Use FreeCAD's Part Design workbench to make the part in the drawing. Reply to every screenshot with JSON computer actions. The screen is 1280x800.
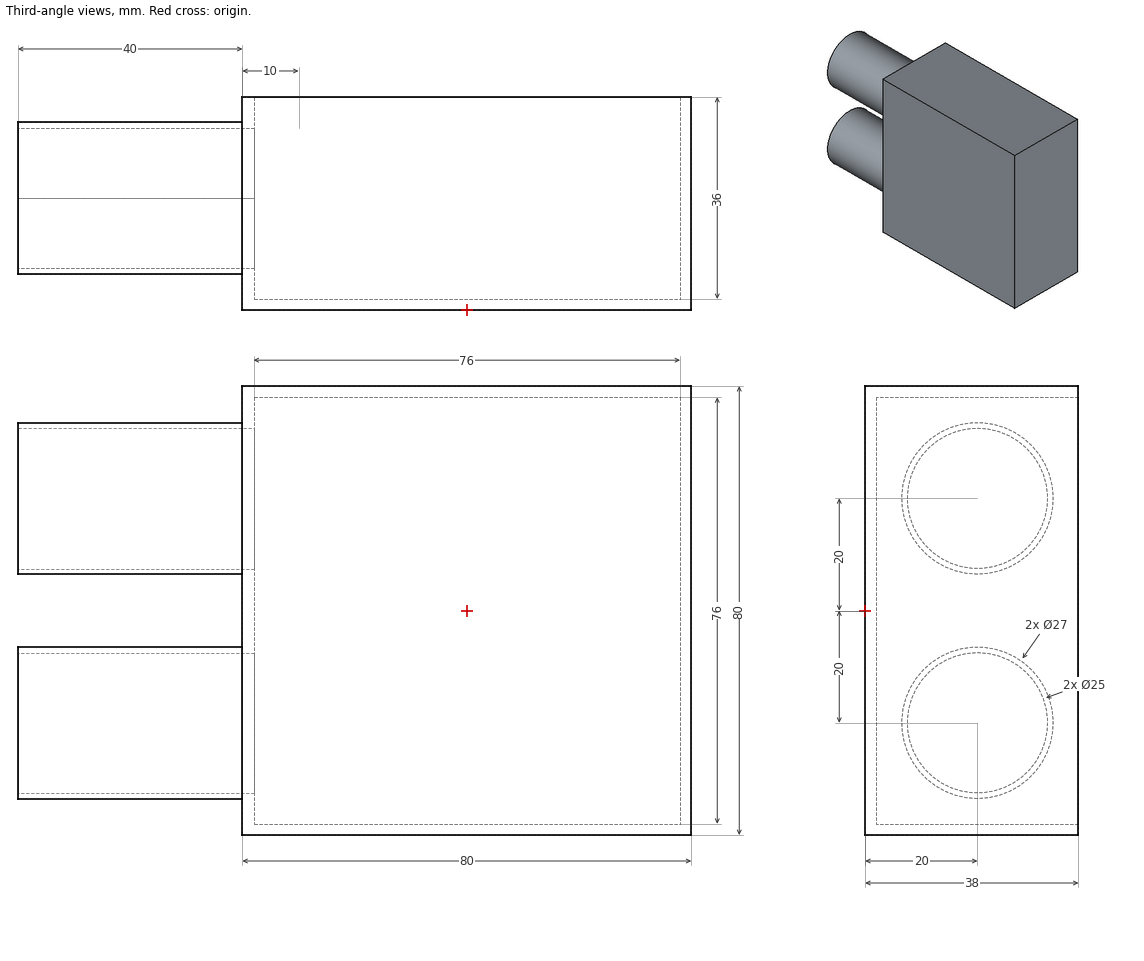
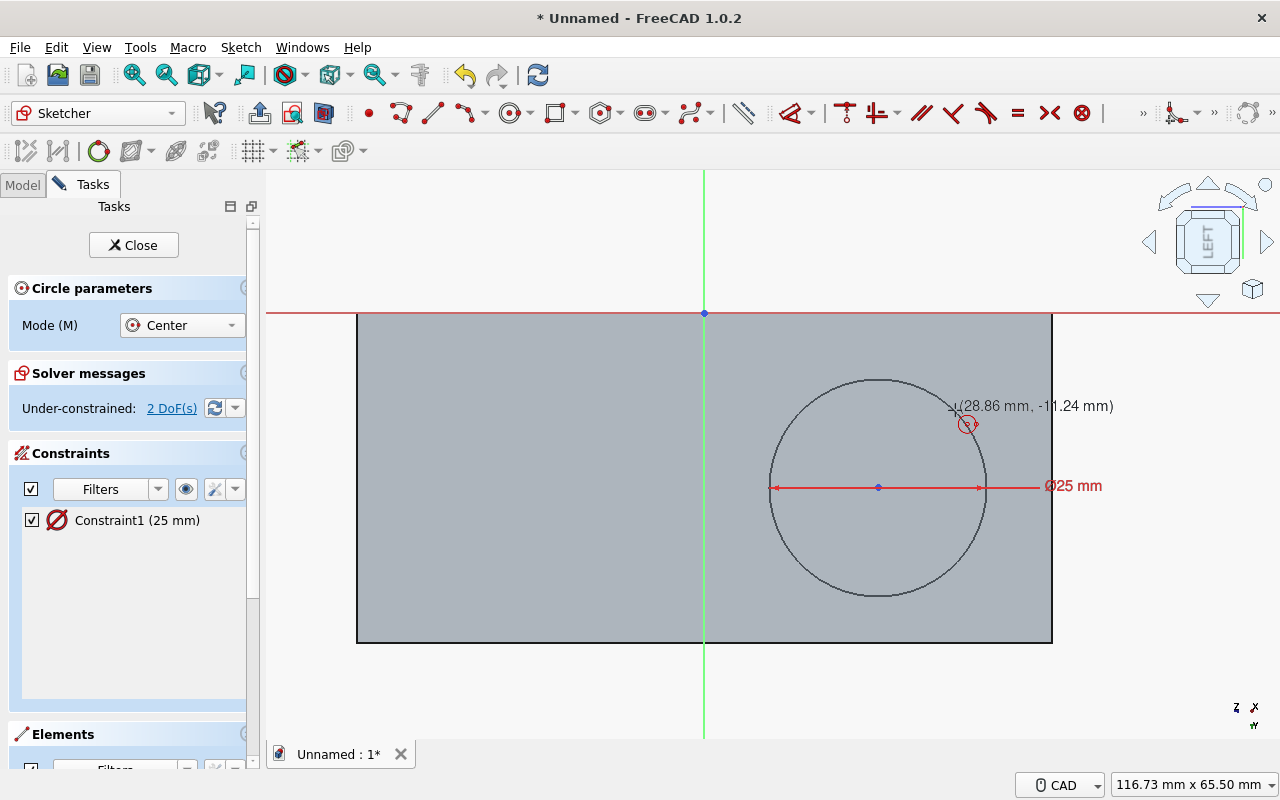
{"action": "left_click", "coordinate": [531, 487]}
{"action": "mouse_move", "coordinate": [607, 410]}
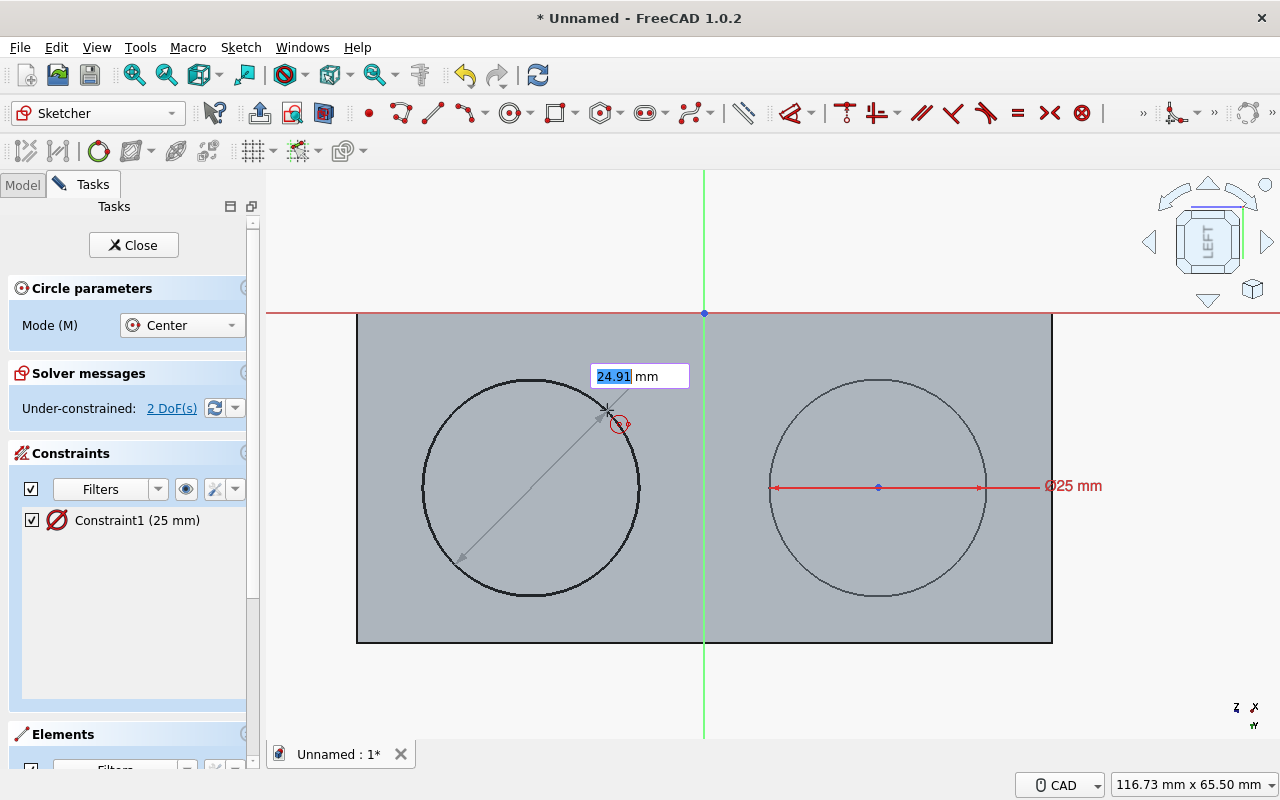
{"action": "type", "text": "25"}
{"action": "key", "text": "Return"}
{"action": "key", "text": "Escape"}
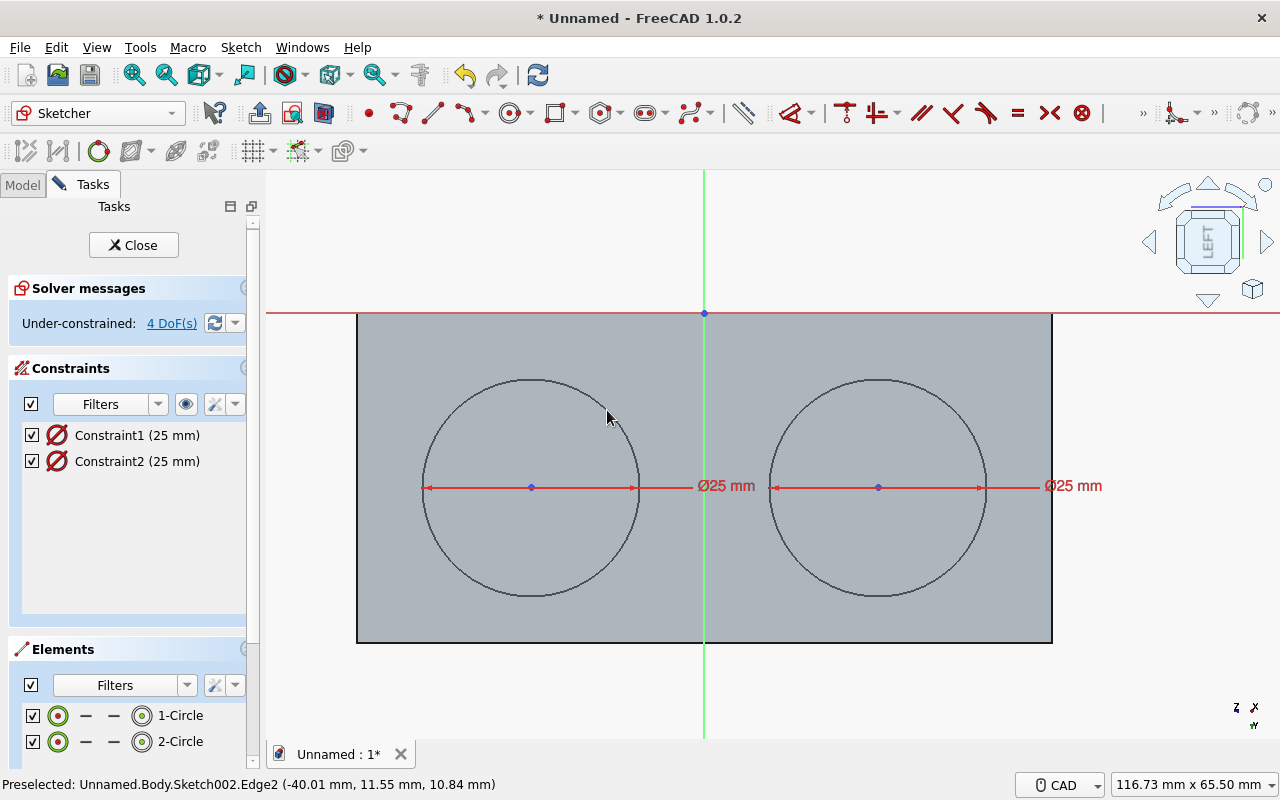
{"action": "left_click", "coordinate": [878, 488]}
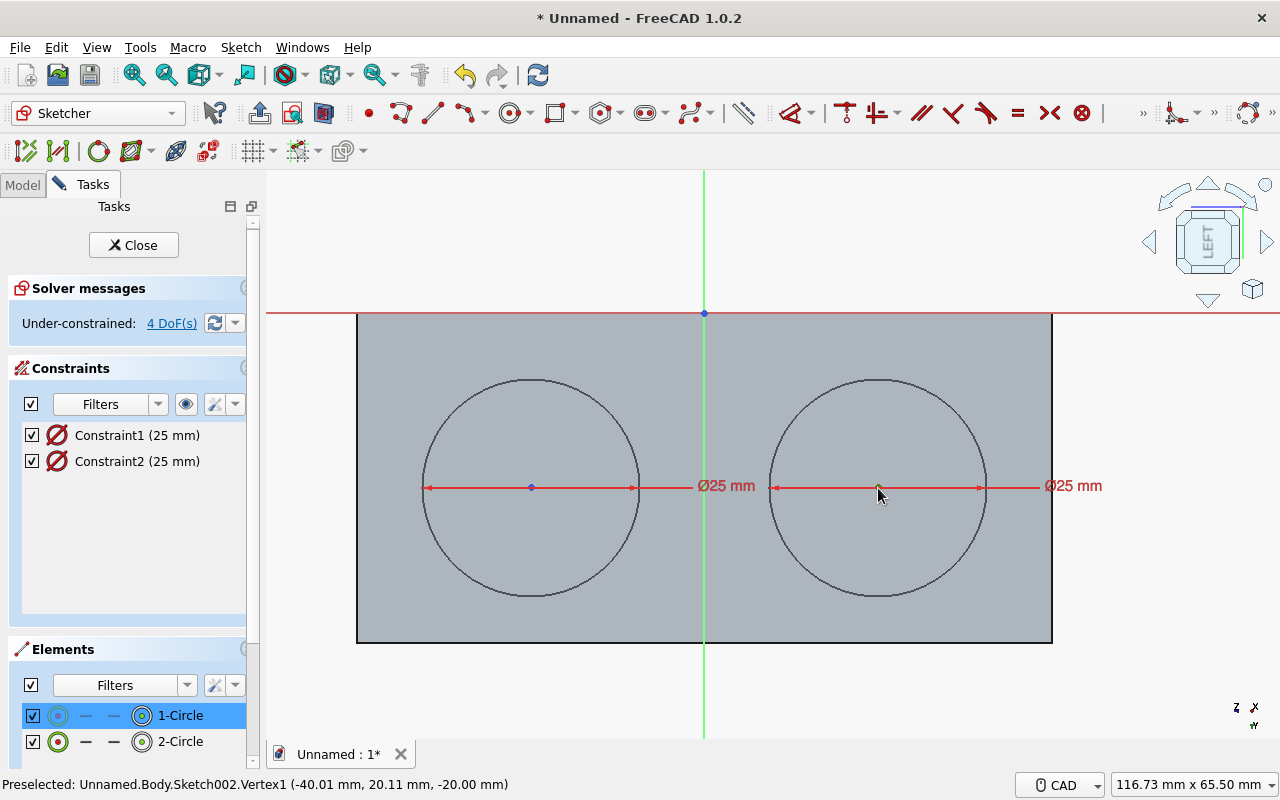
{"action": "left_click", "coordinate": [531, 488]}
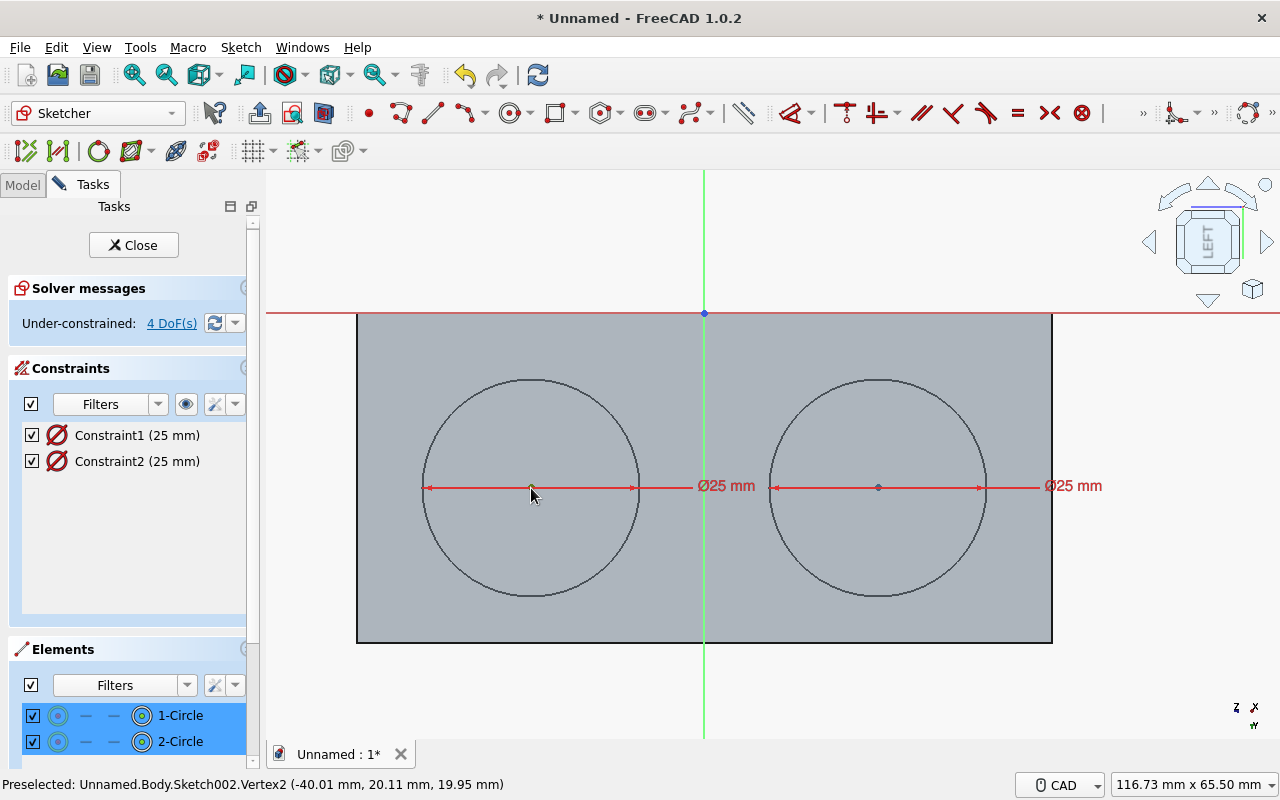
{"action": "left_click", "coordinate": [900, 114]}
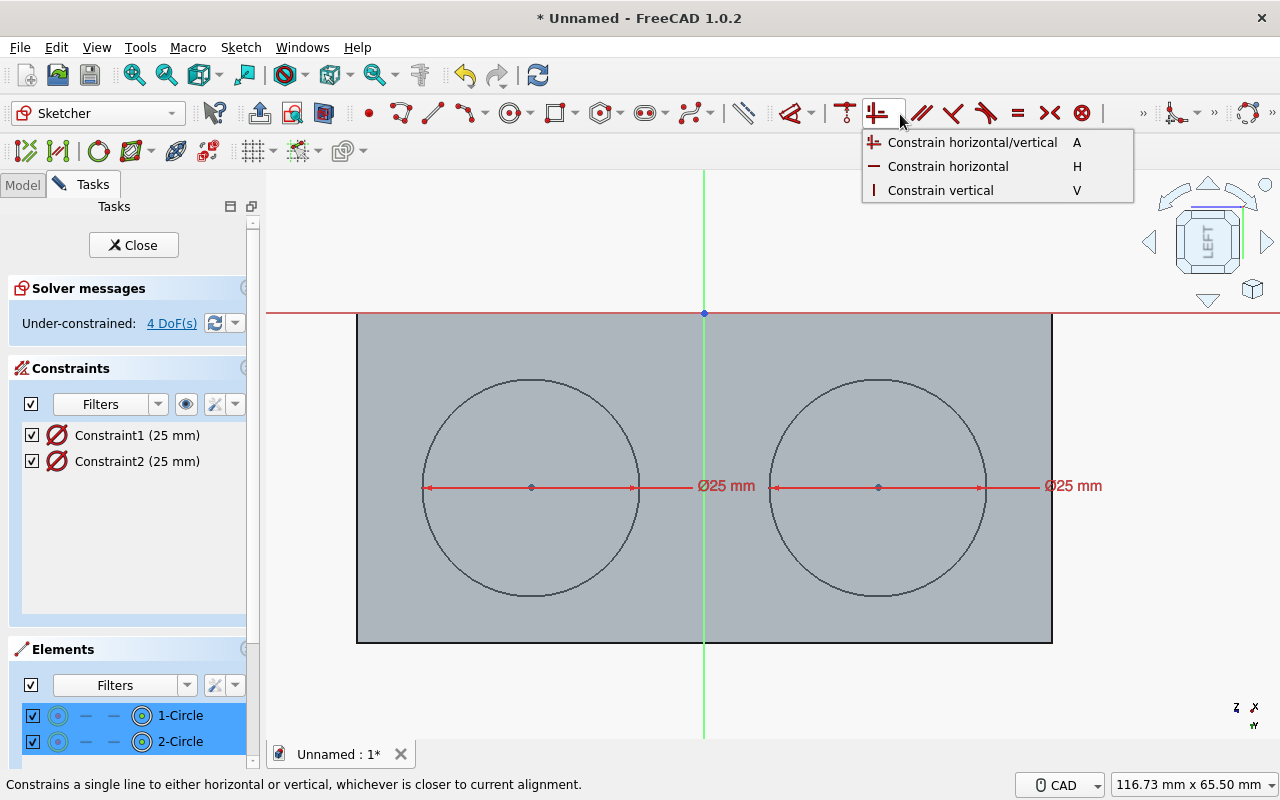
{"action": "left_click", "coordinate": [998, 166]}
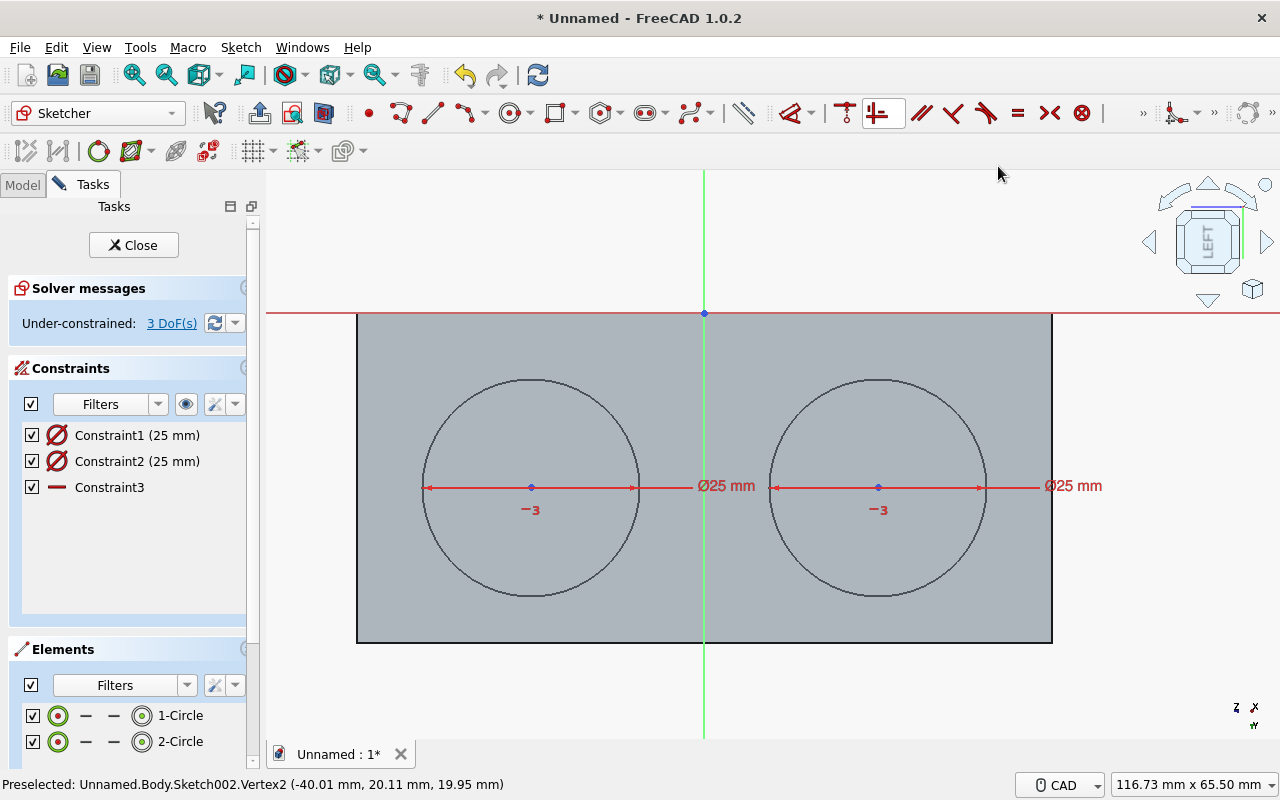
{"action": "left_click", "coordinate": [790, 114]}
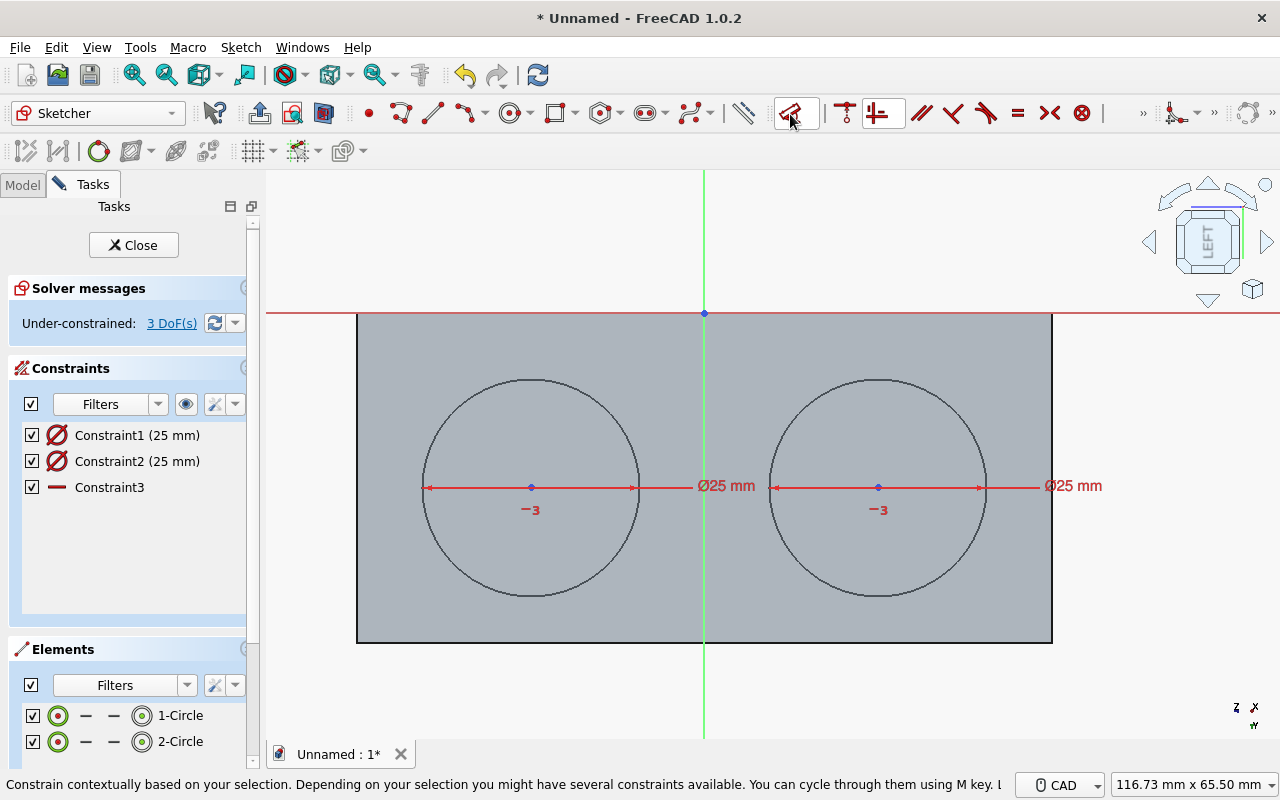
{"action": "left_click", "coordinate": [878, 488]}
{"action": "left_click", "coordinate": [791, 279]}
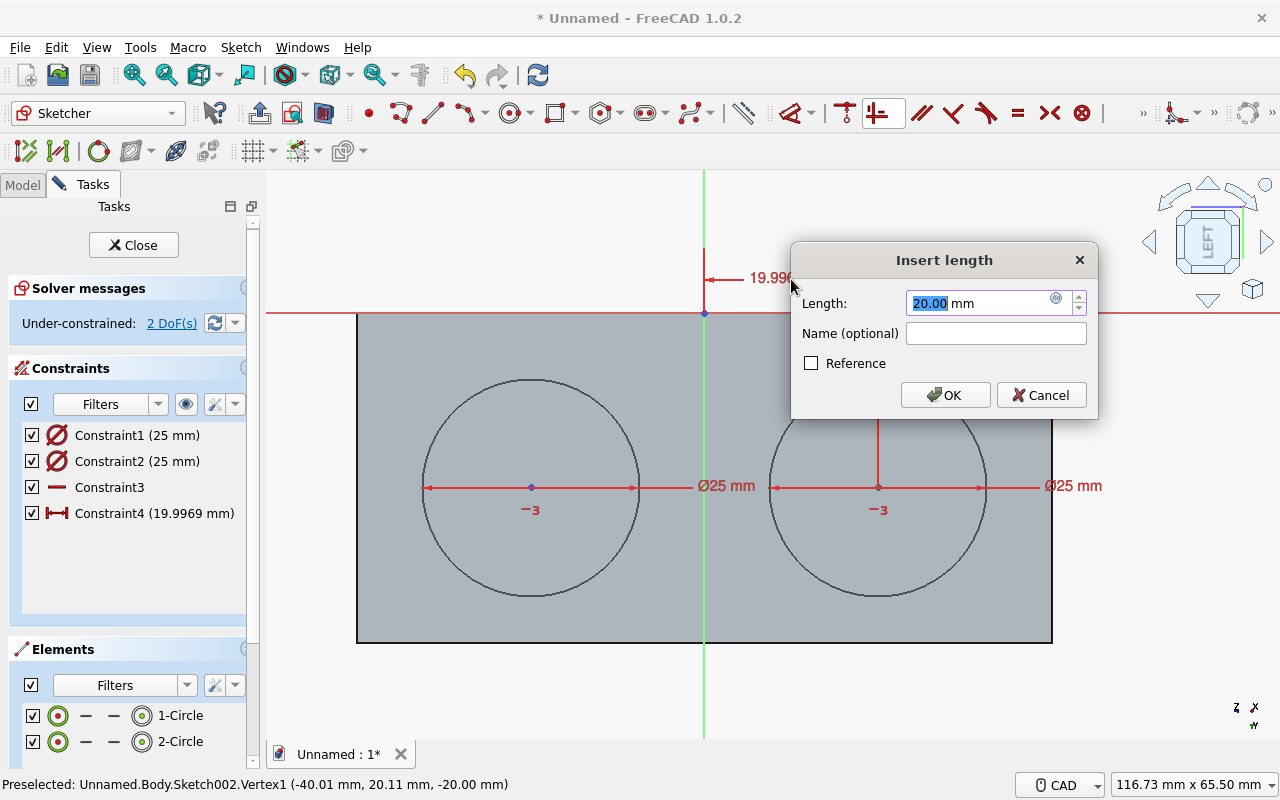
{"action": "type", "text": "20"}
{"action": "key", "text": "Return"}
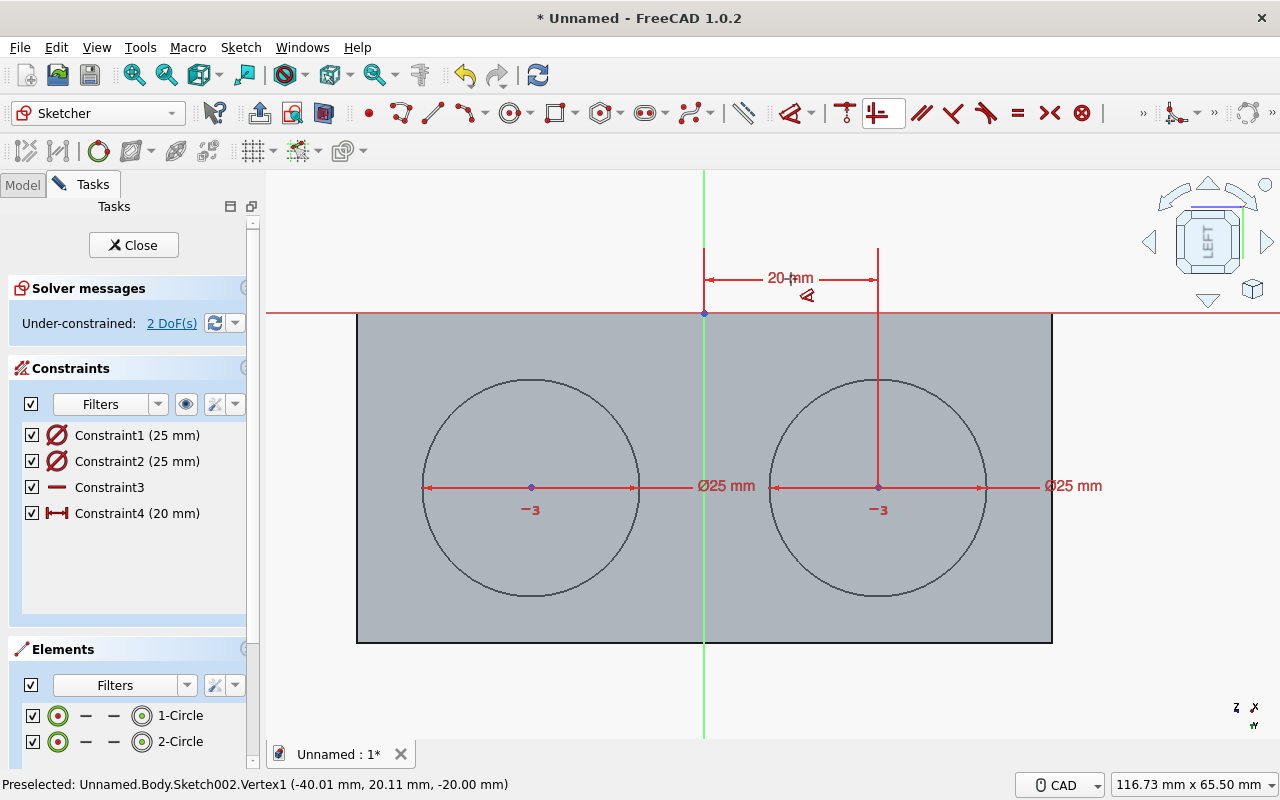
{"action": "left_click", "coordinate": [878, 488]}
{"action": "left_click", "coordinate": [912, 401]}